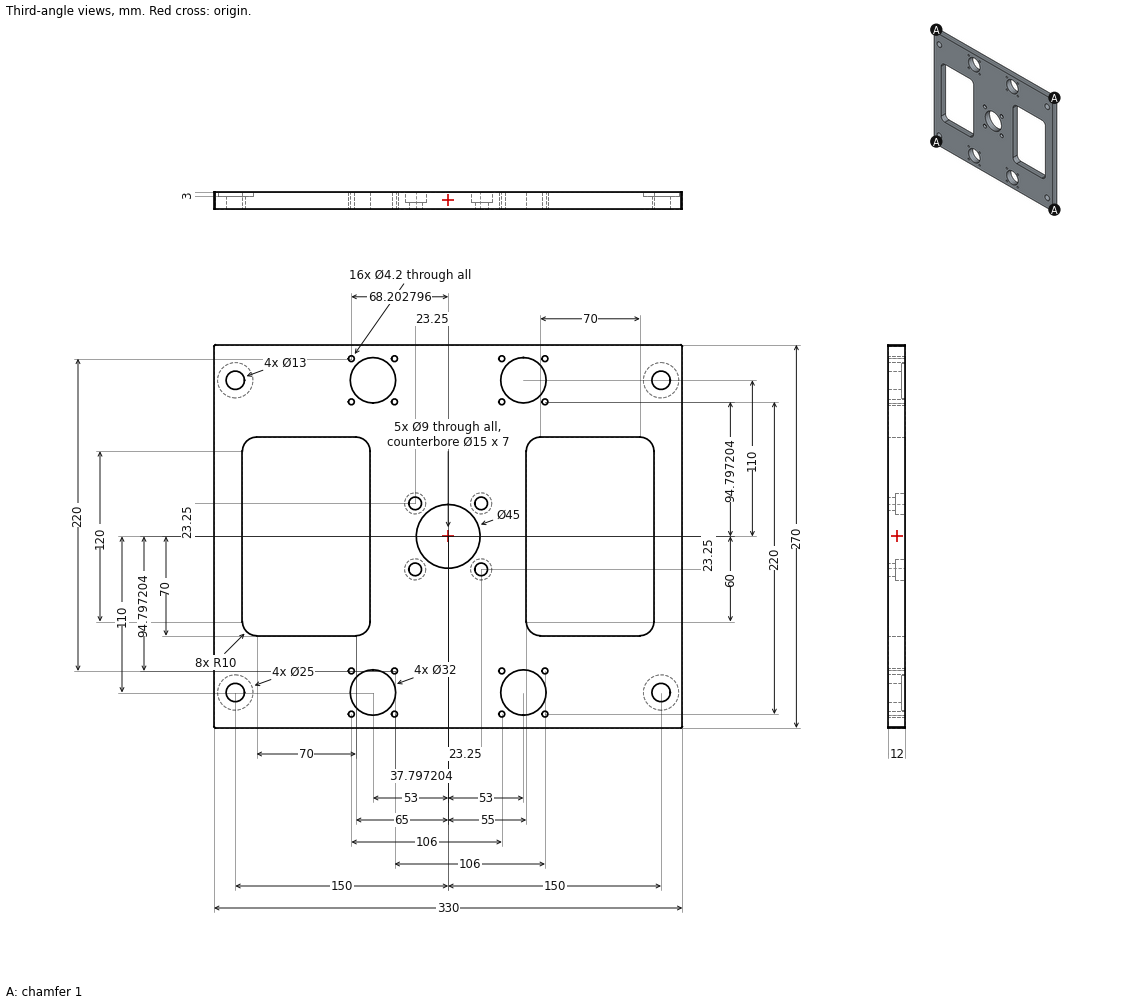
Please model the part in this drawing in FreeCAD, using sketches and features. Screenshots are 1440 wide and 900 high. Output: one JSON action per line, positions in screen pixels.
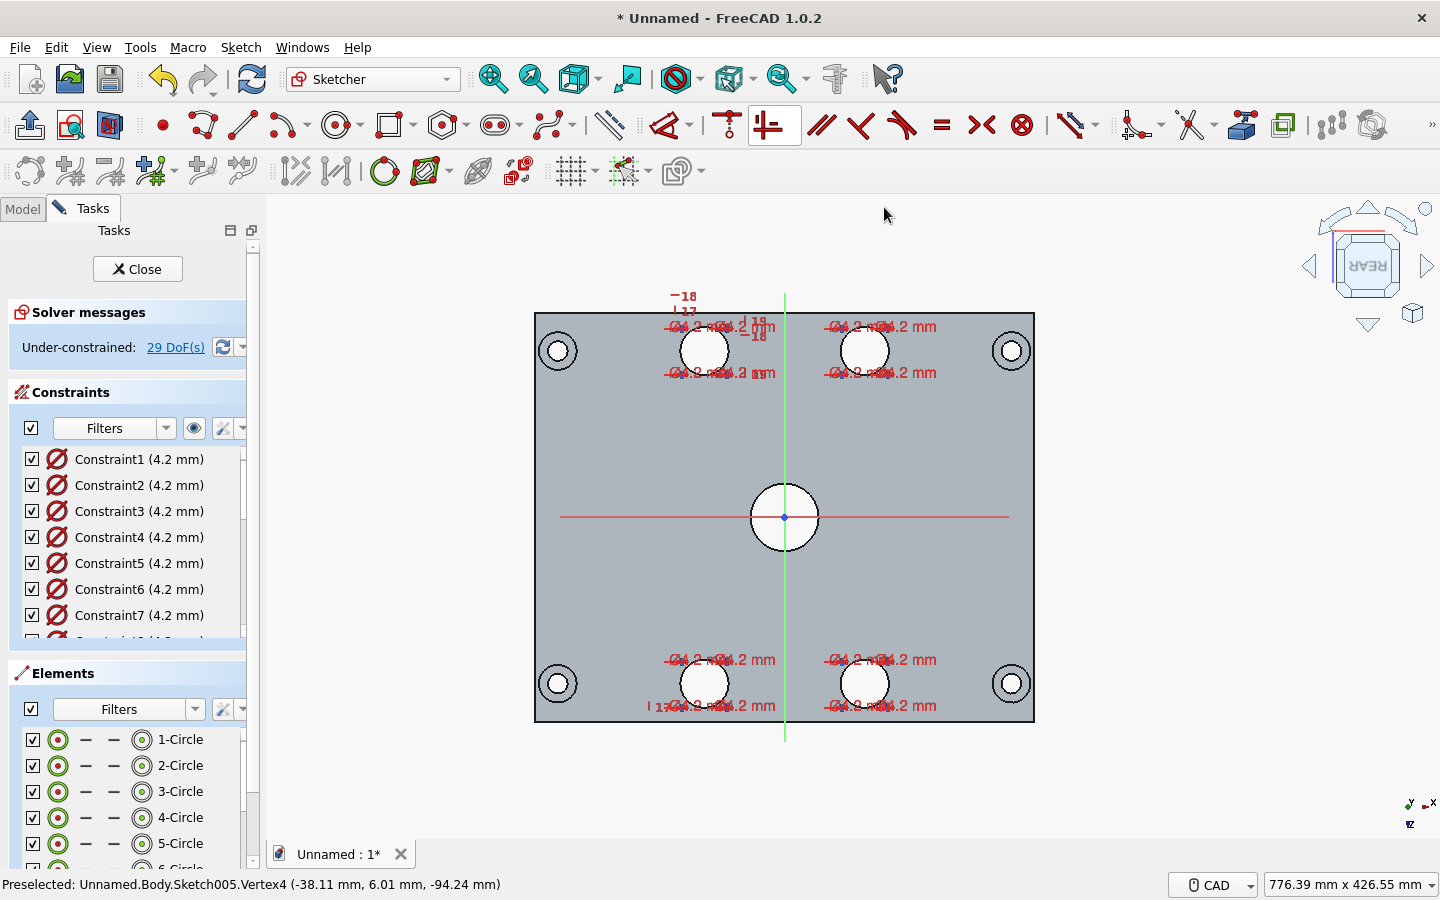
{"action": "left_click", "coordinate": [682, 329]}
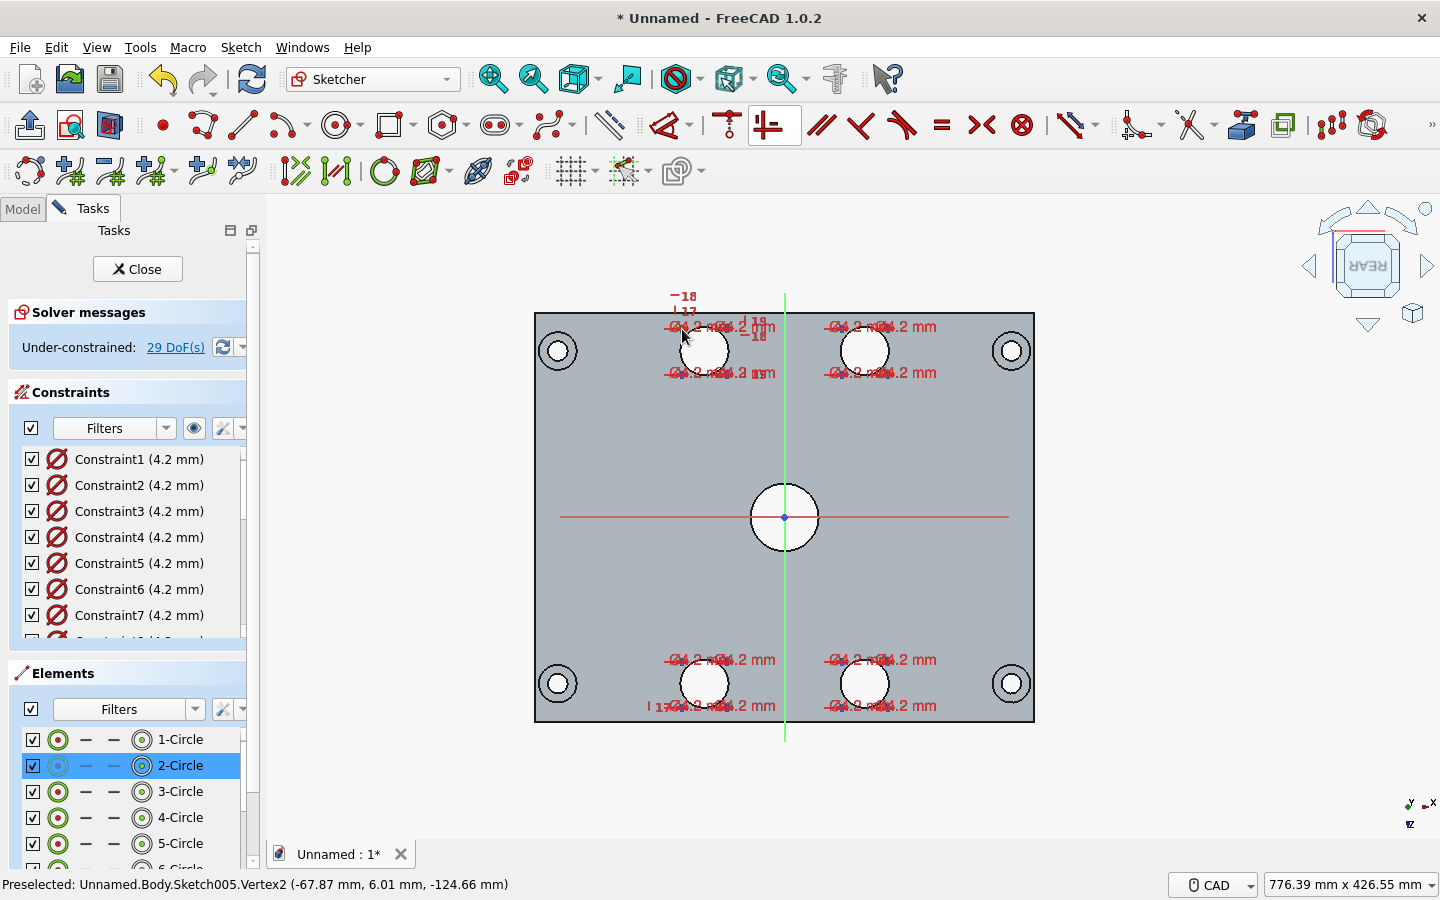
{"action": "left_click", "coordinate": [682, 375]}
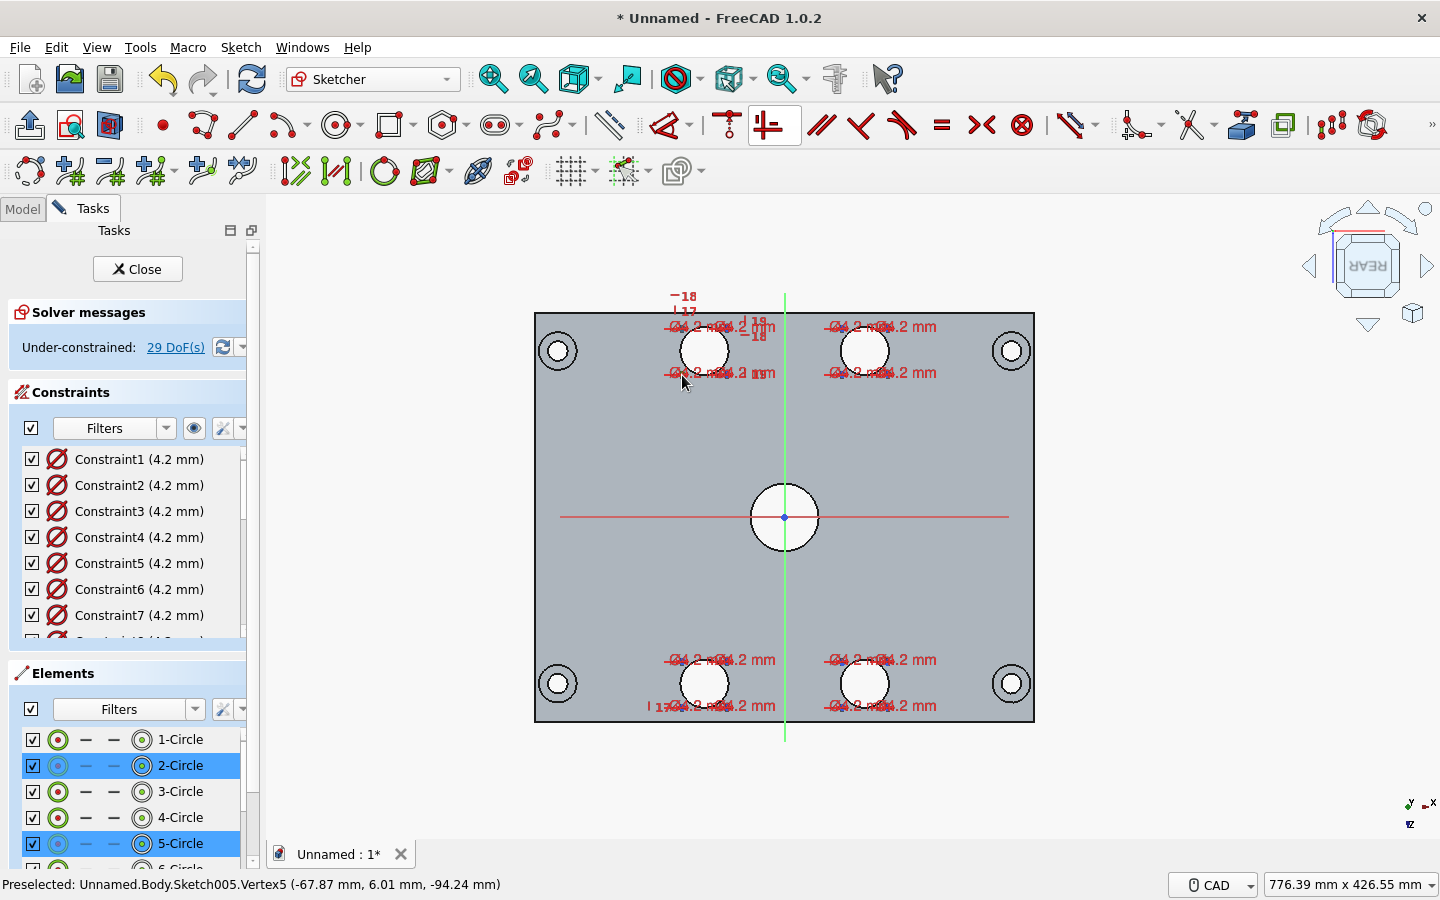
{"action": "key", "text": "v"}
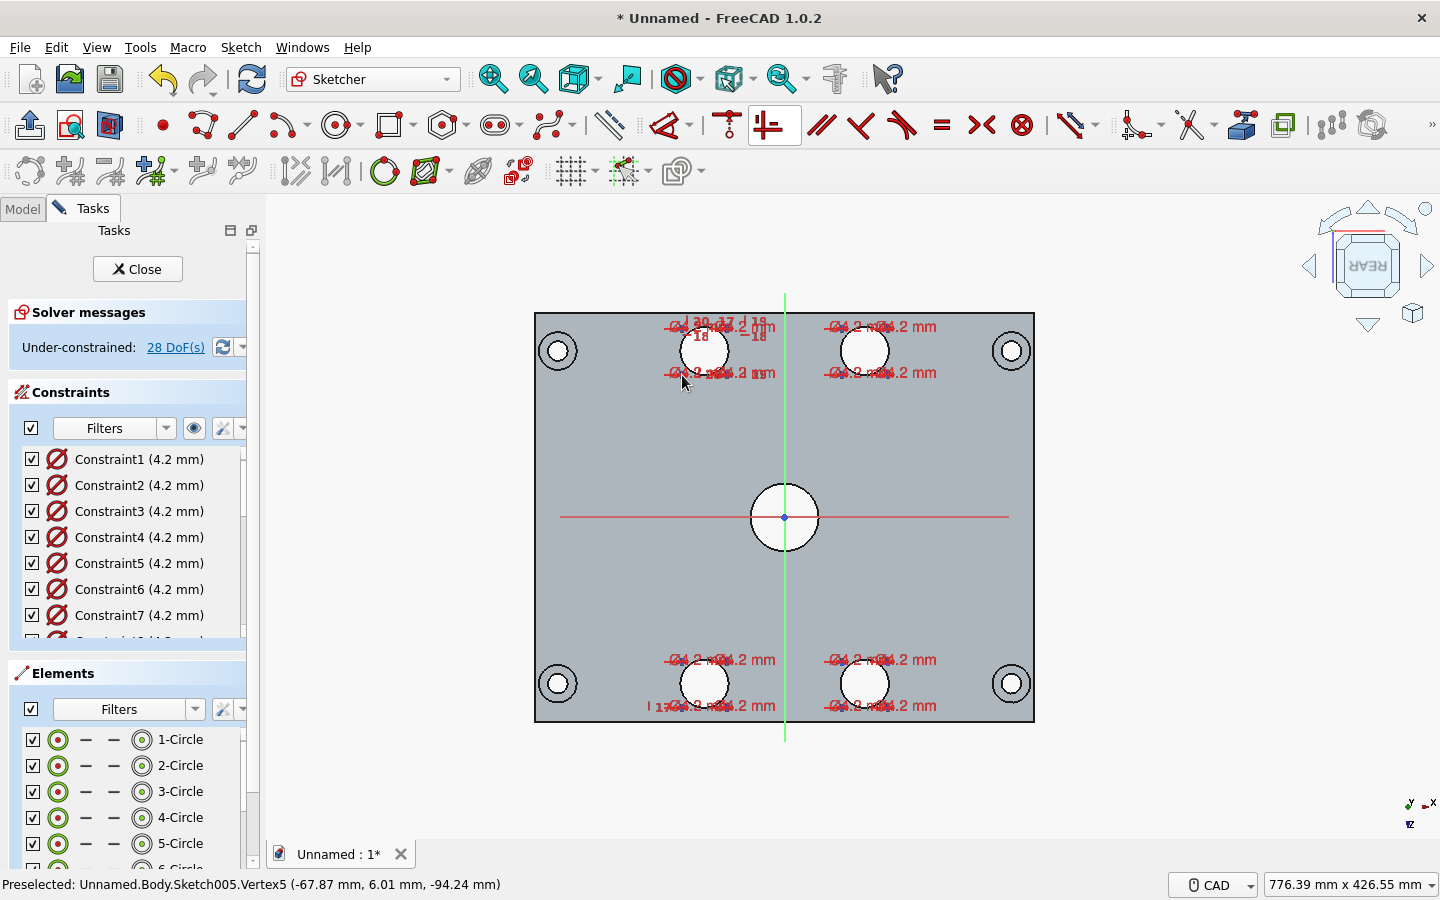
{"action": "left_click", "coordinate": [727, 375]}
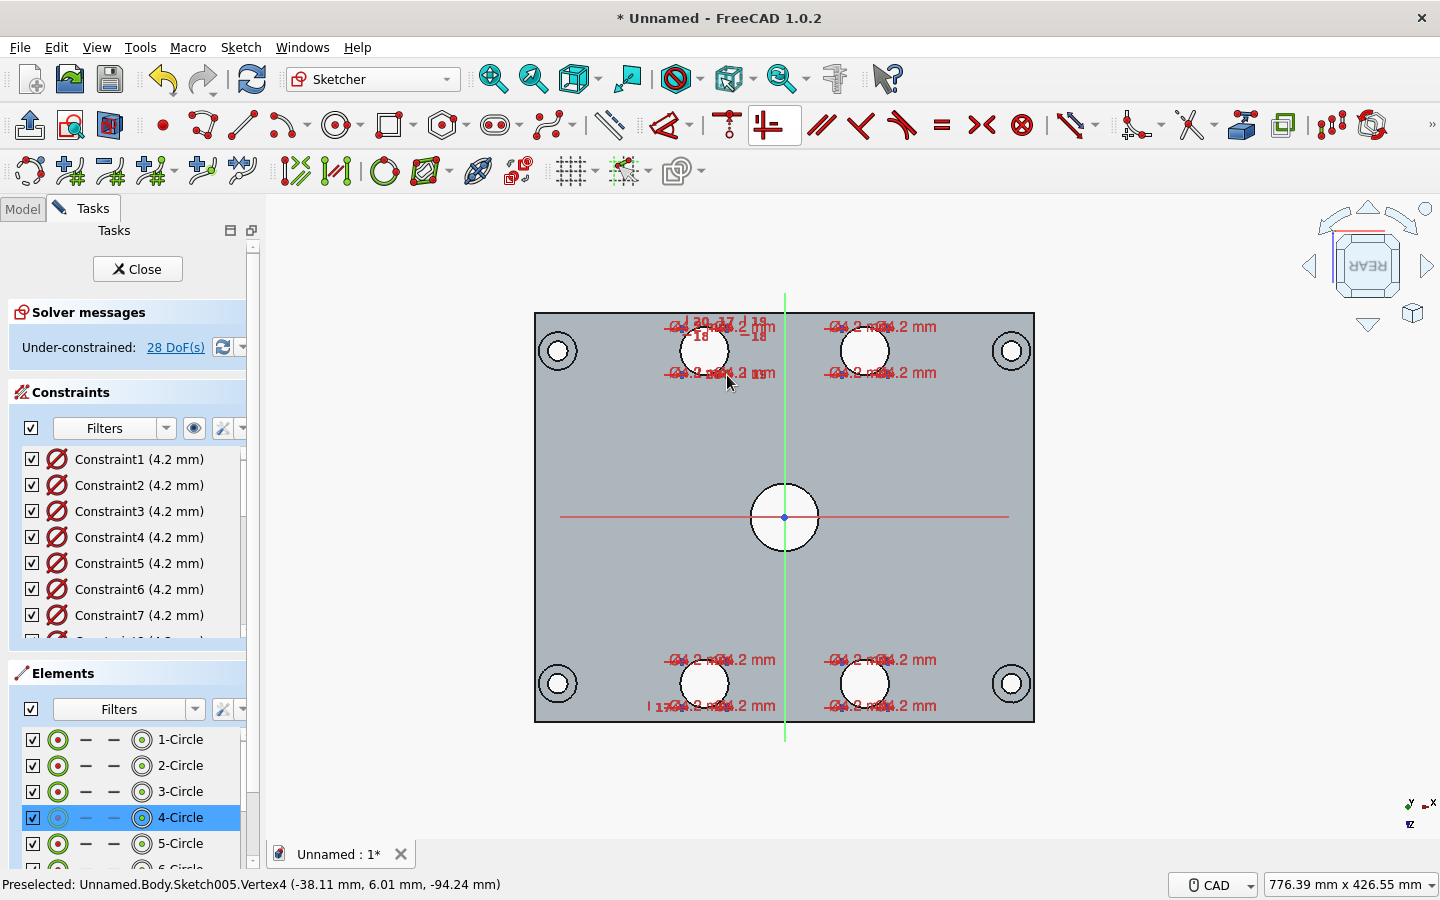
{"action": "left_click", "coordinate": [682, 375]}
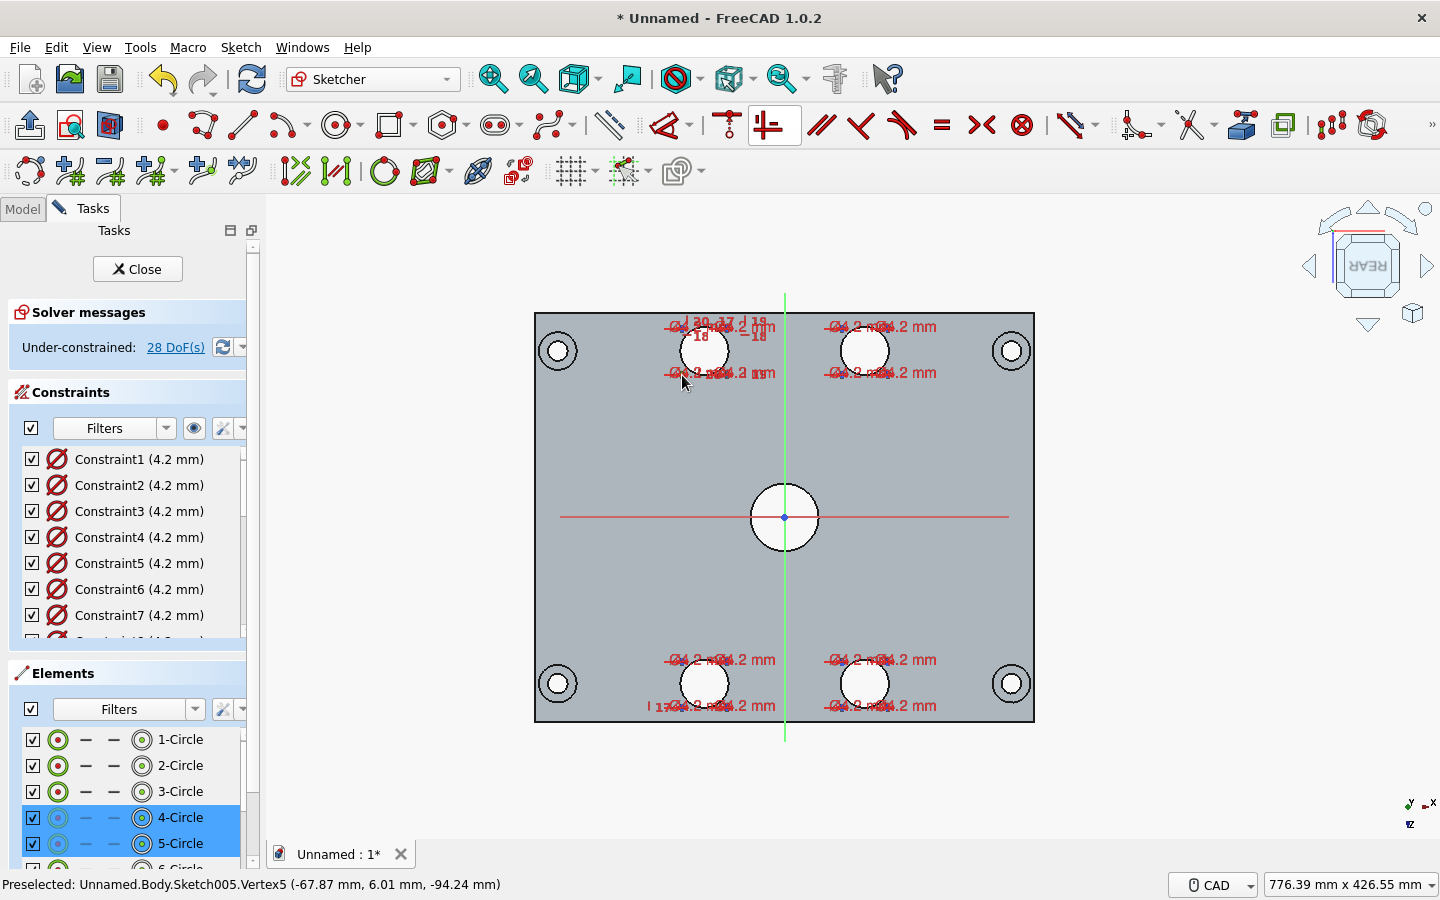
{"action": "key", "text": "h"}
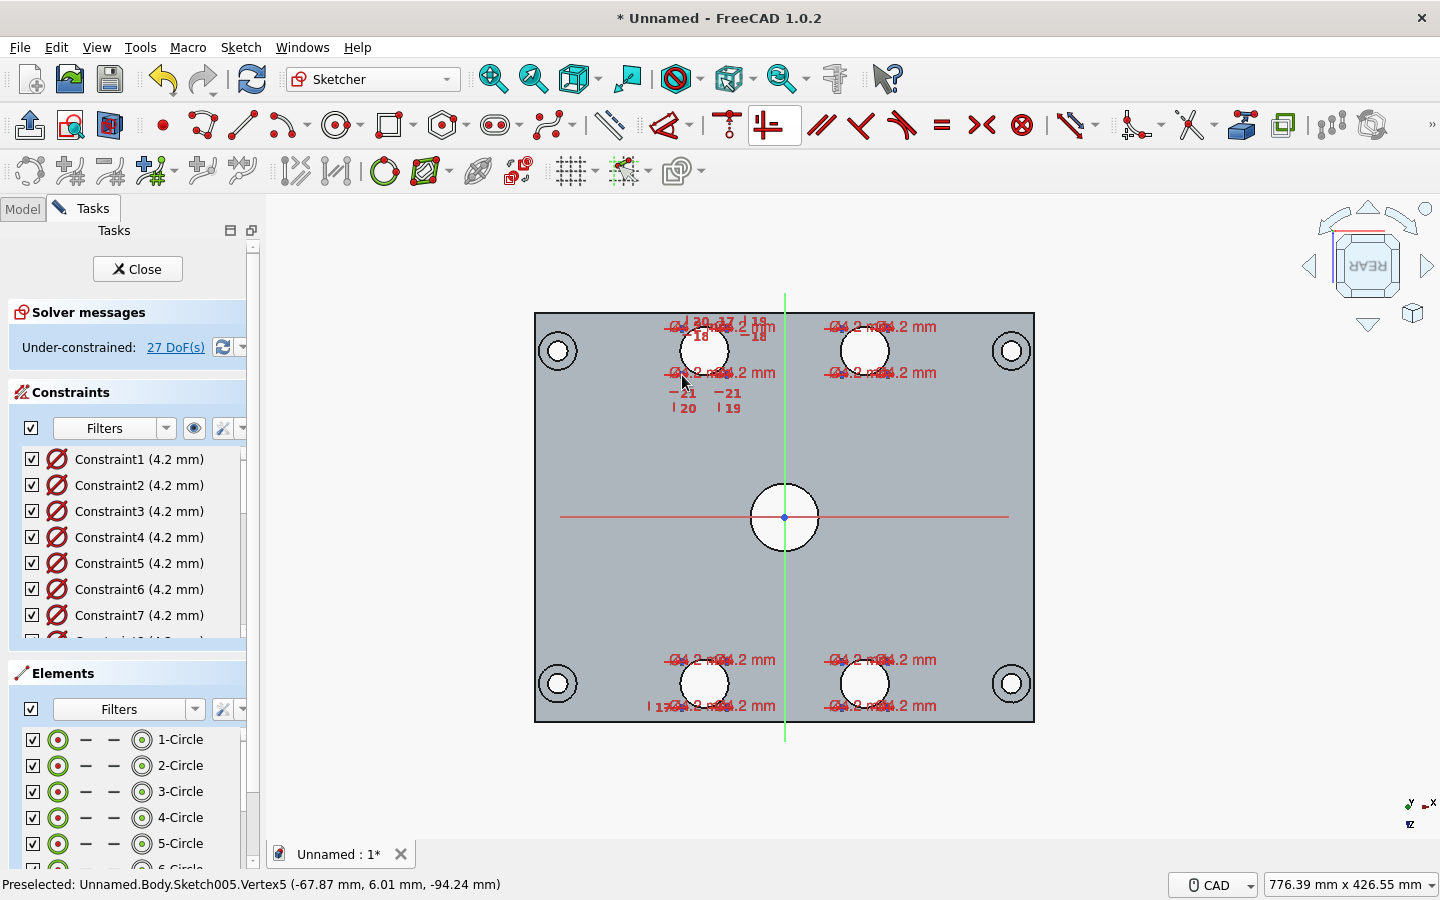
{"action": "left_click", "coordinate": [727, 329]}